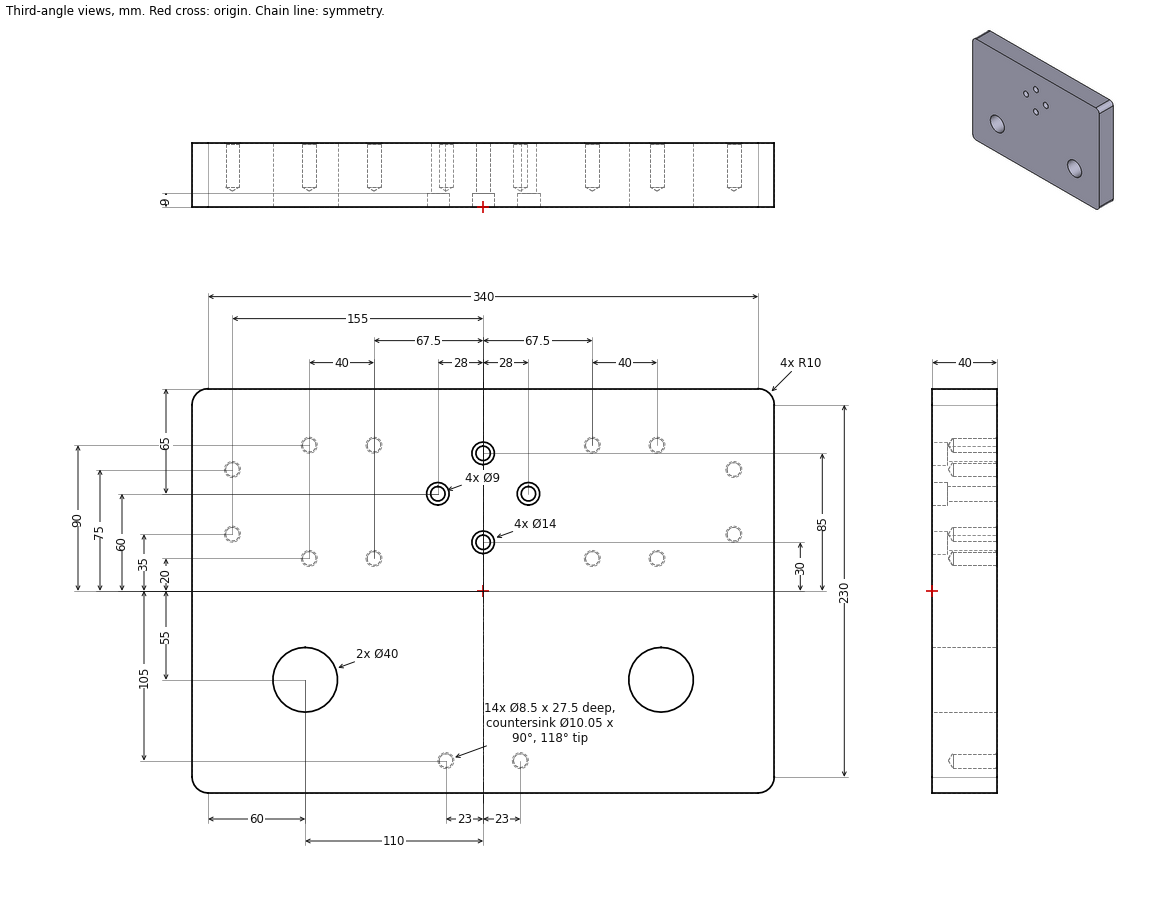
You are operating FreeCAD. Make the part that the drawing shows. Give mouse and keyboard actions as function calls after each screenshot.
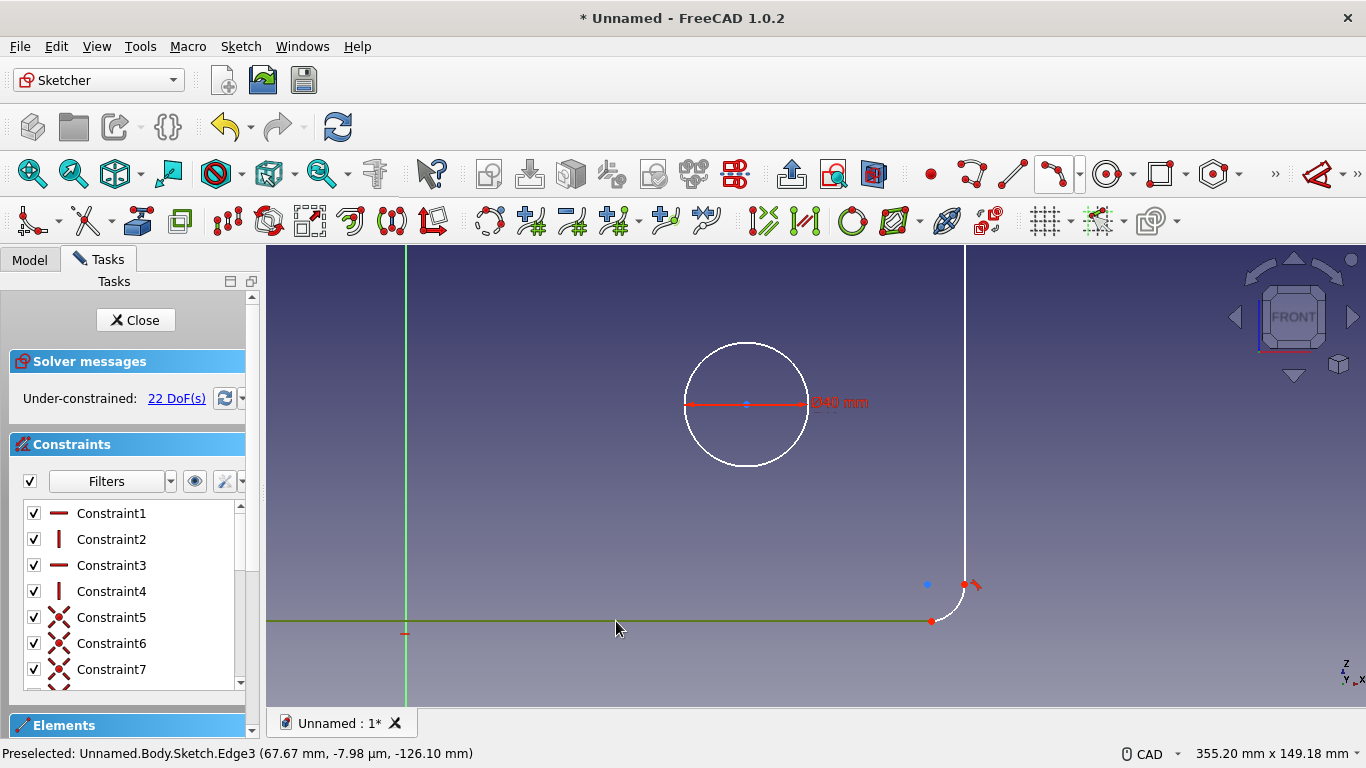
click(947, 616)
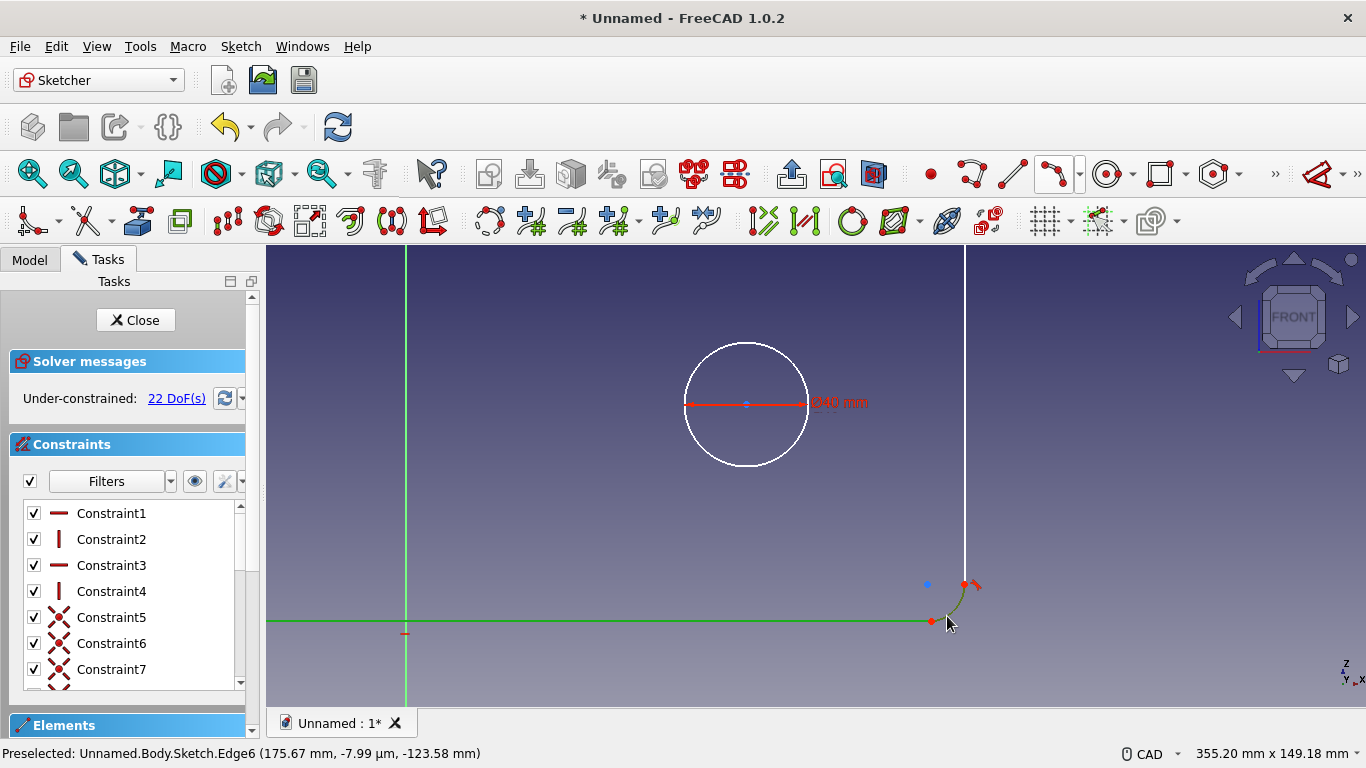
key(t)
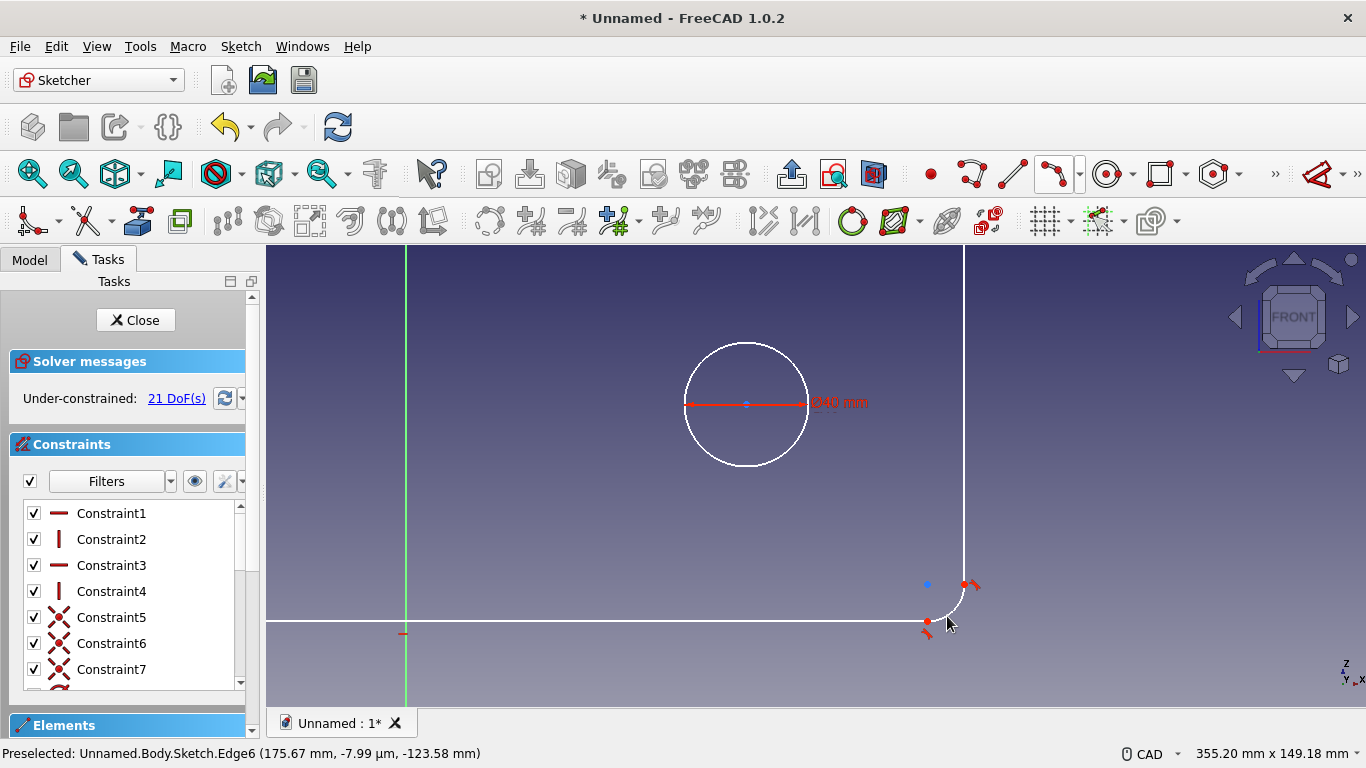
click(613, 621)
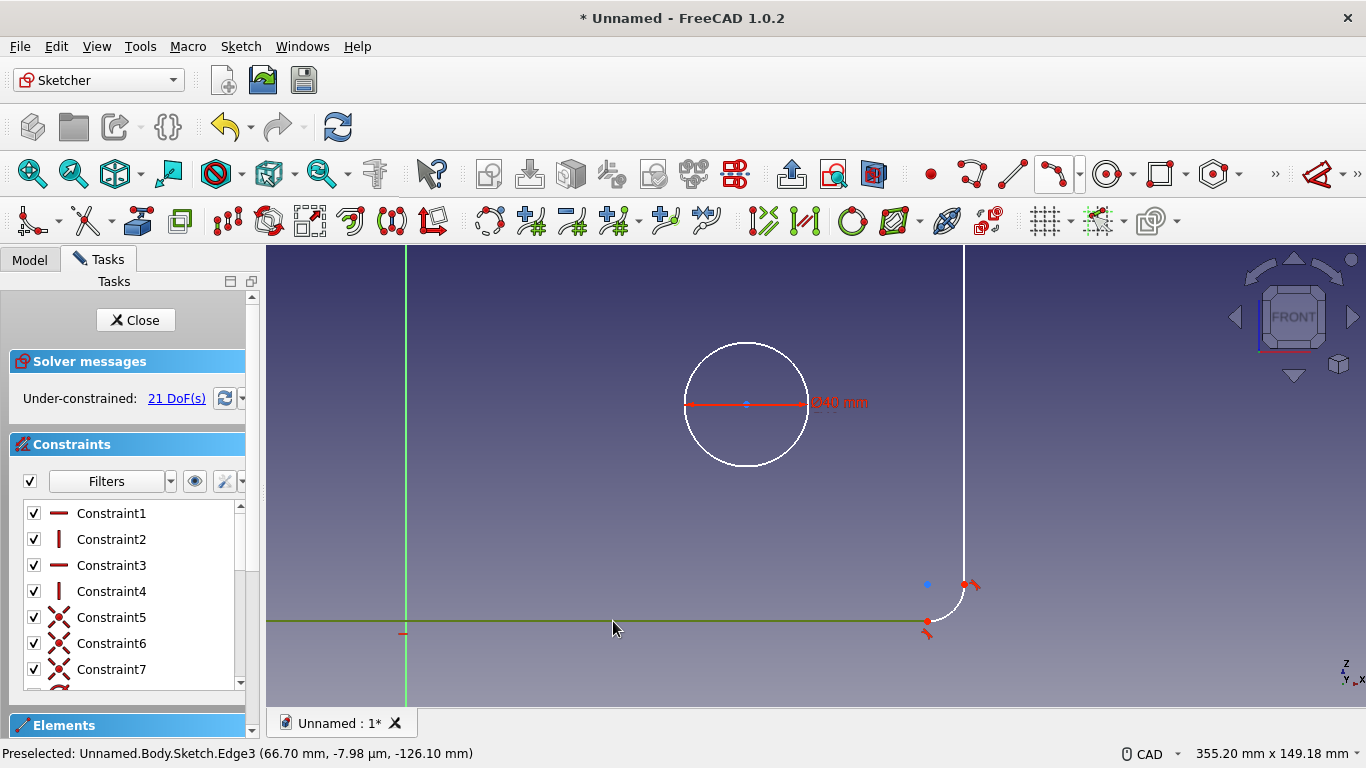
scroll(946, 619, down, 5)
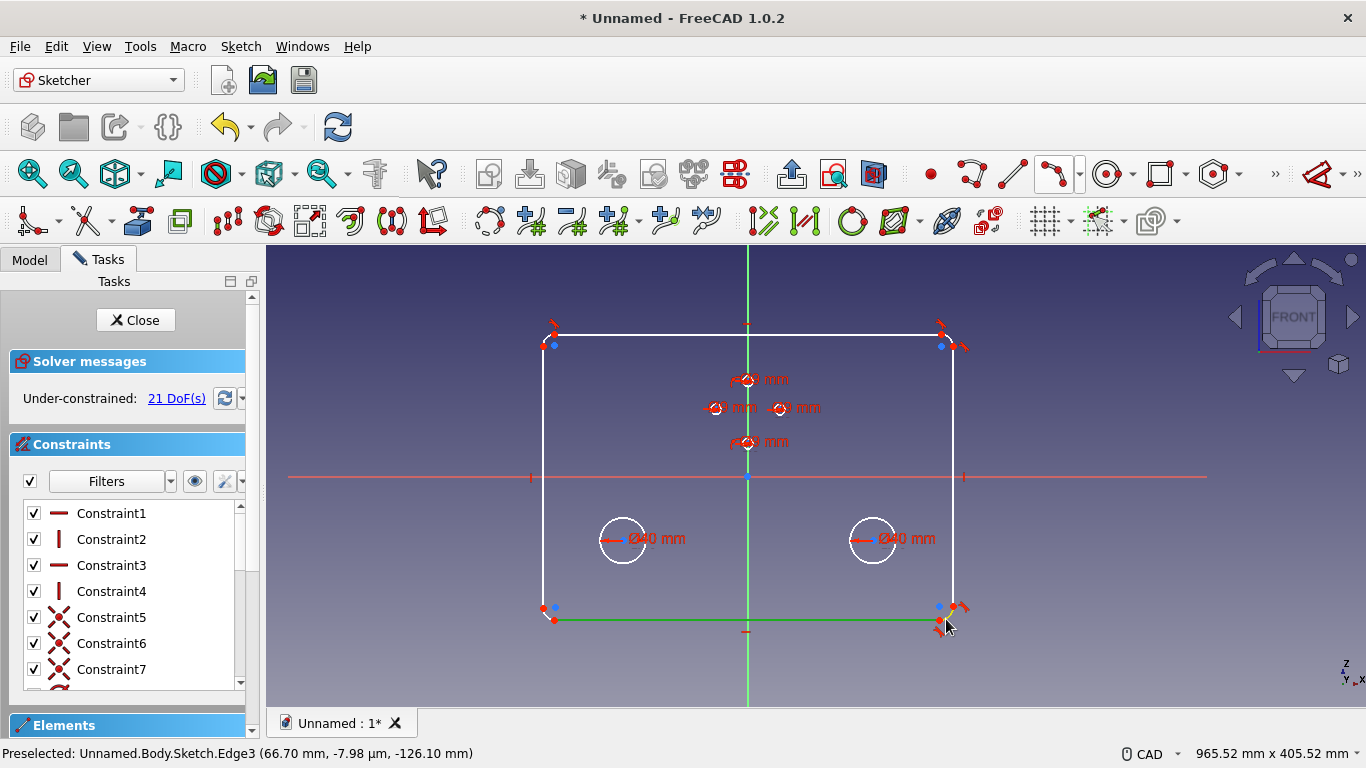
scroll(544, 613, up, 5)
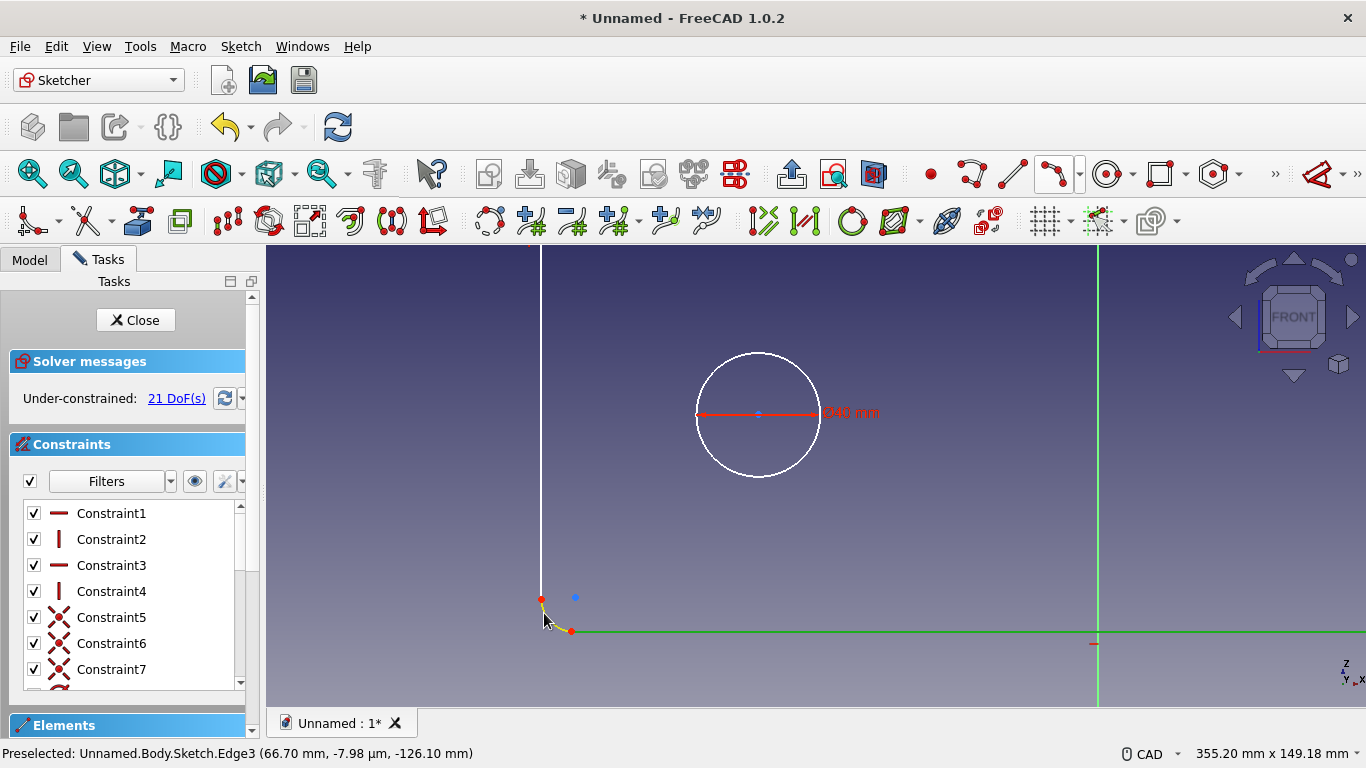
click(545, 613)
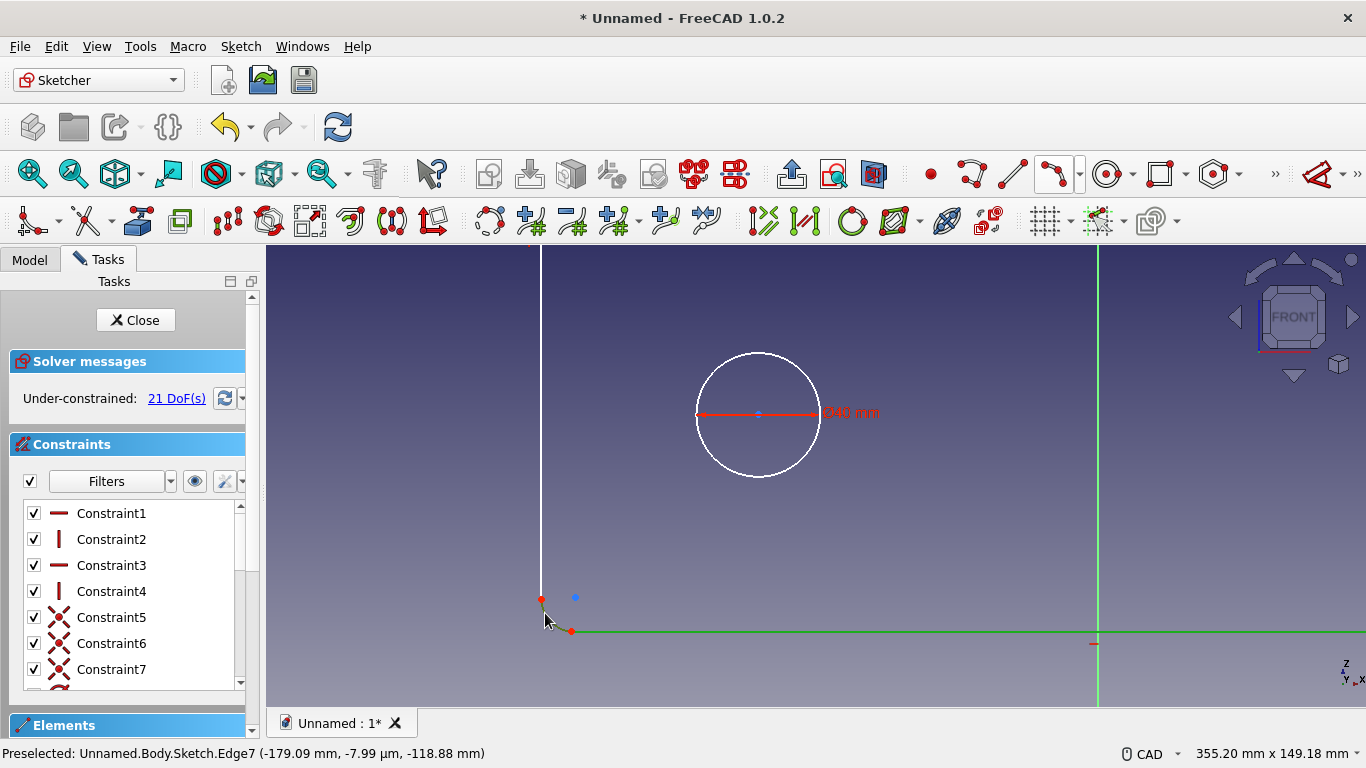
key(t)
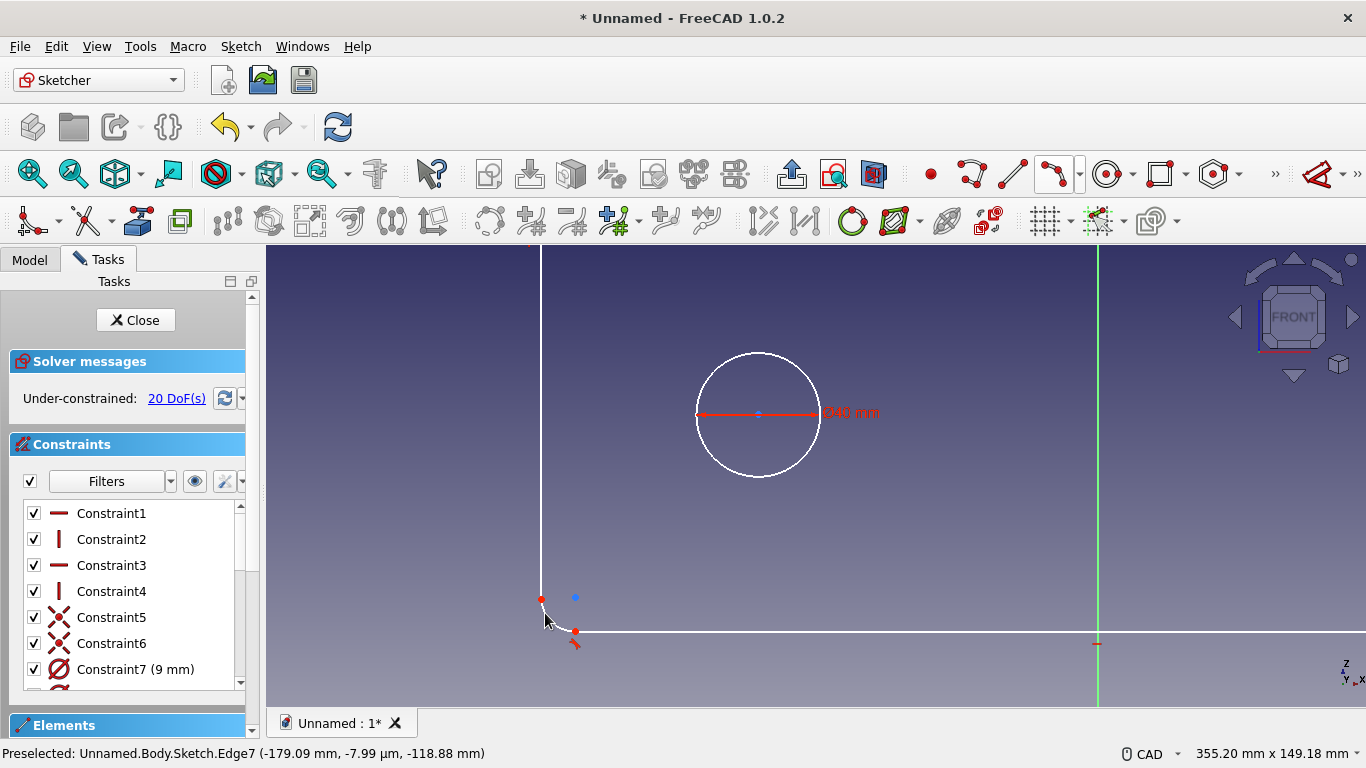
click(541, 385)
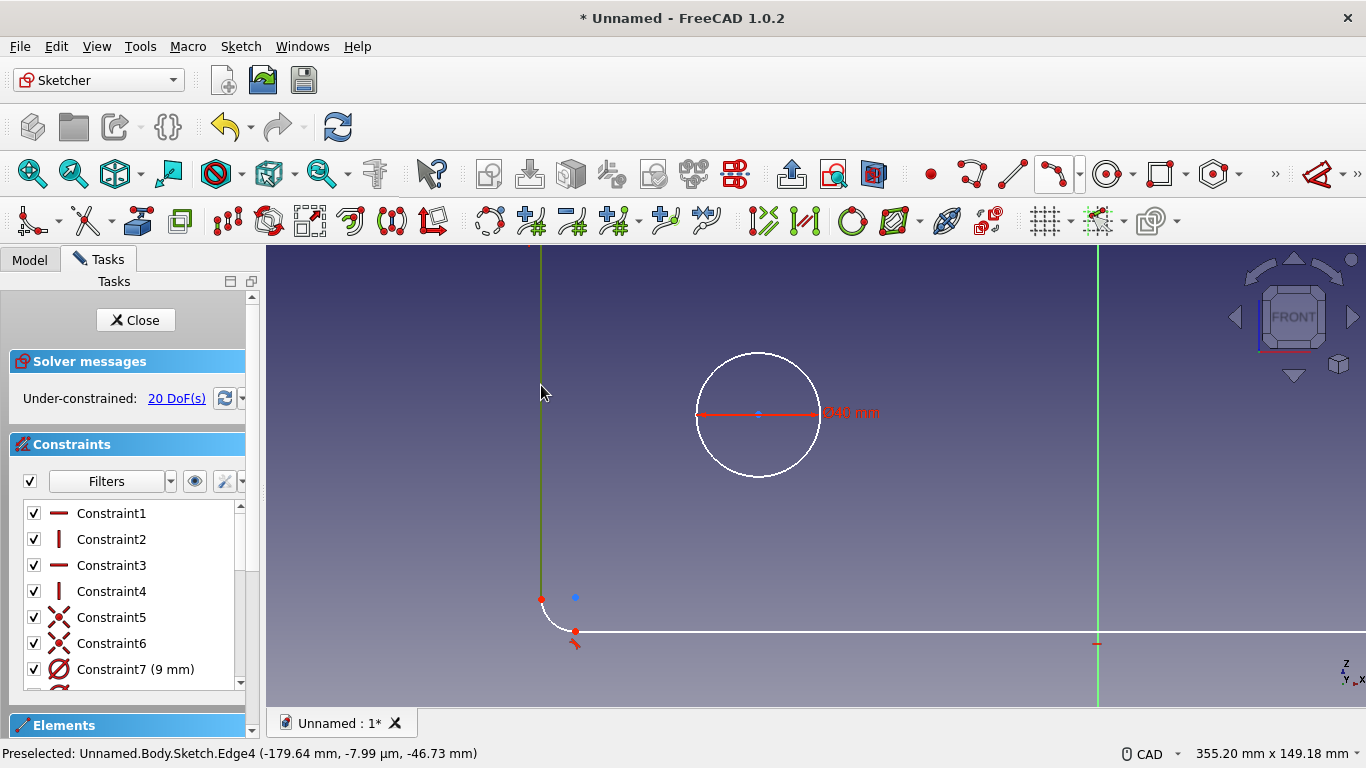
click(546, 614)